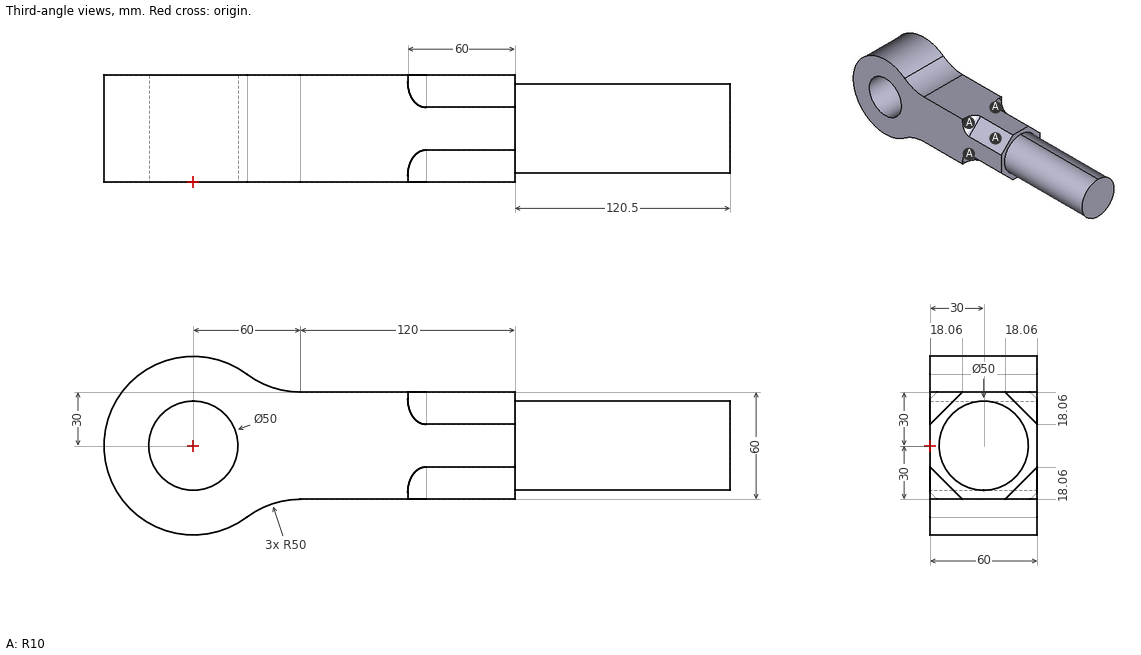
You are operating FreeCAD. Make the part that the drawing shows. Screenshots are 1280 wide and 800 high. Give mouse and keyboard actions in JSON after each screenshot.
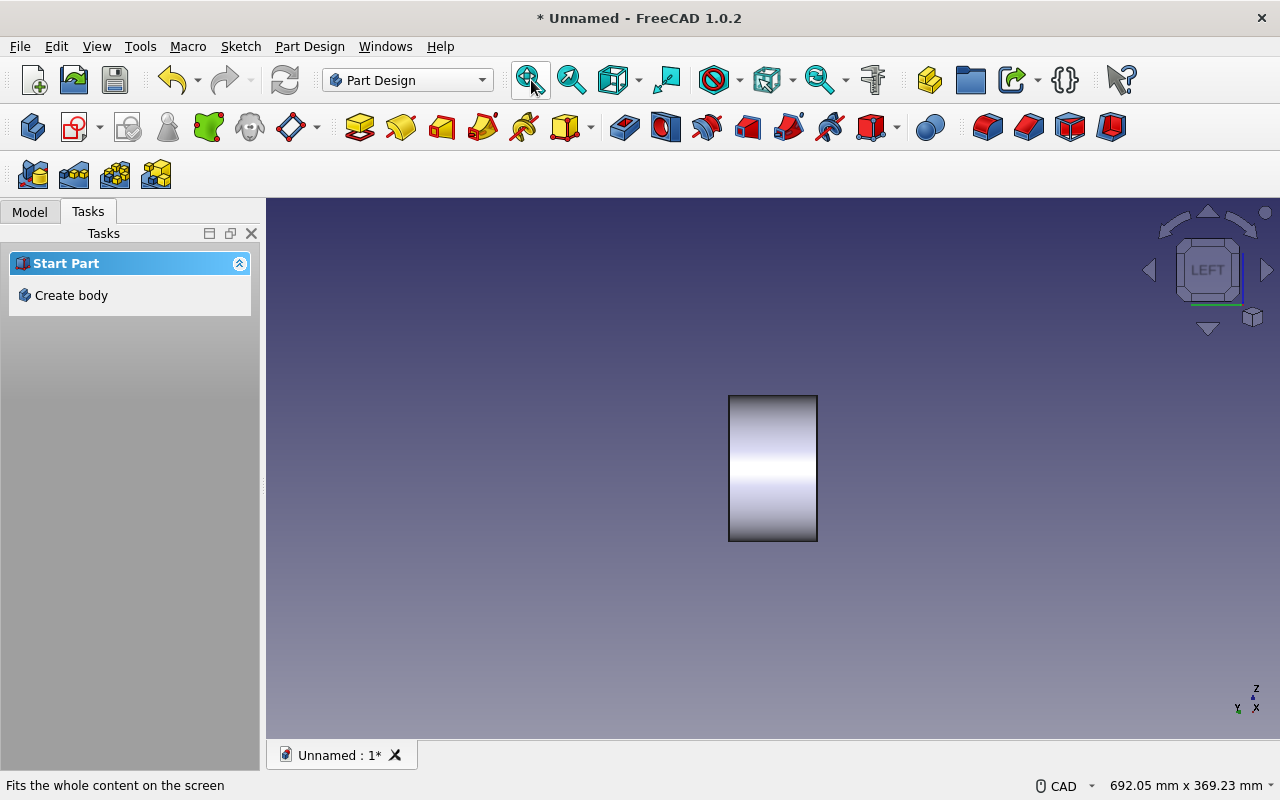
{"action": "key", "text": "v 3"}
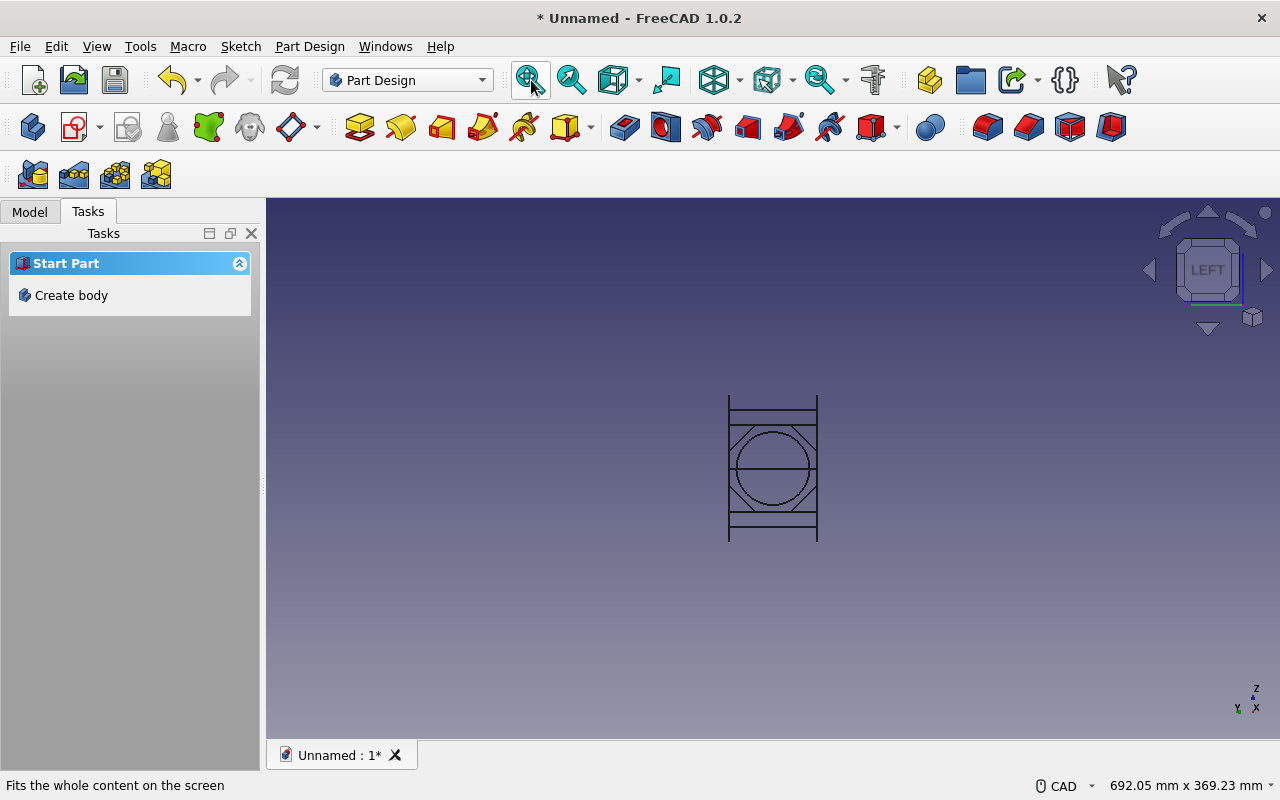
{"action": "key", "text": "0"}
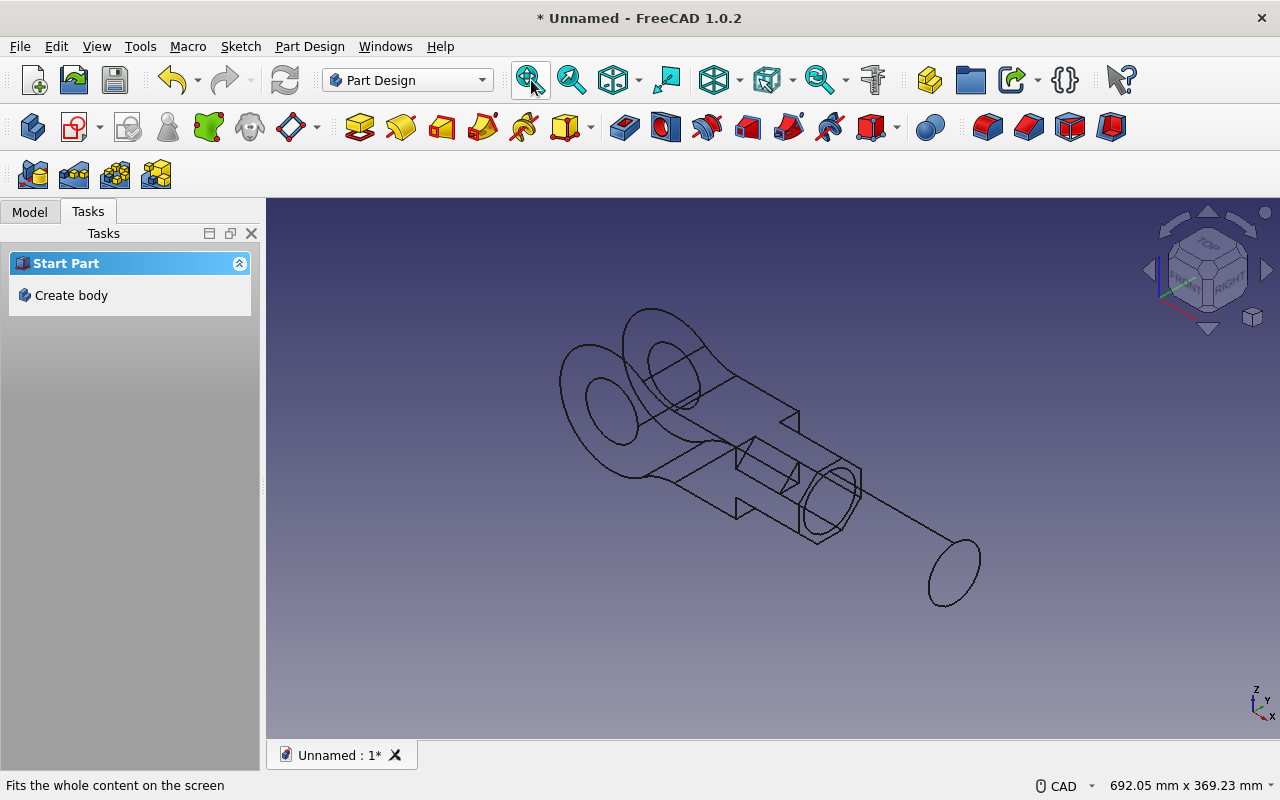
{"action": "left_click", "coordinate": [789, 477]}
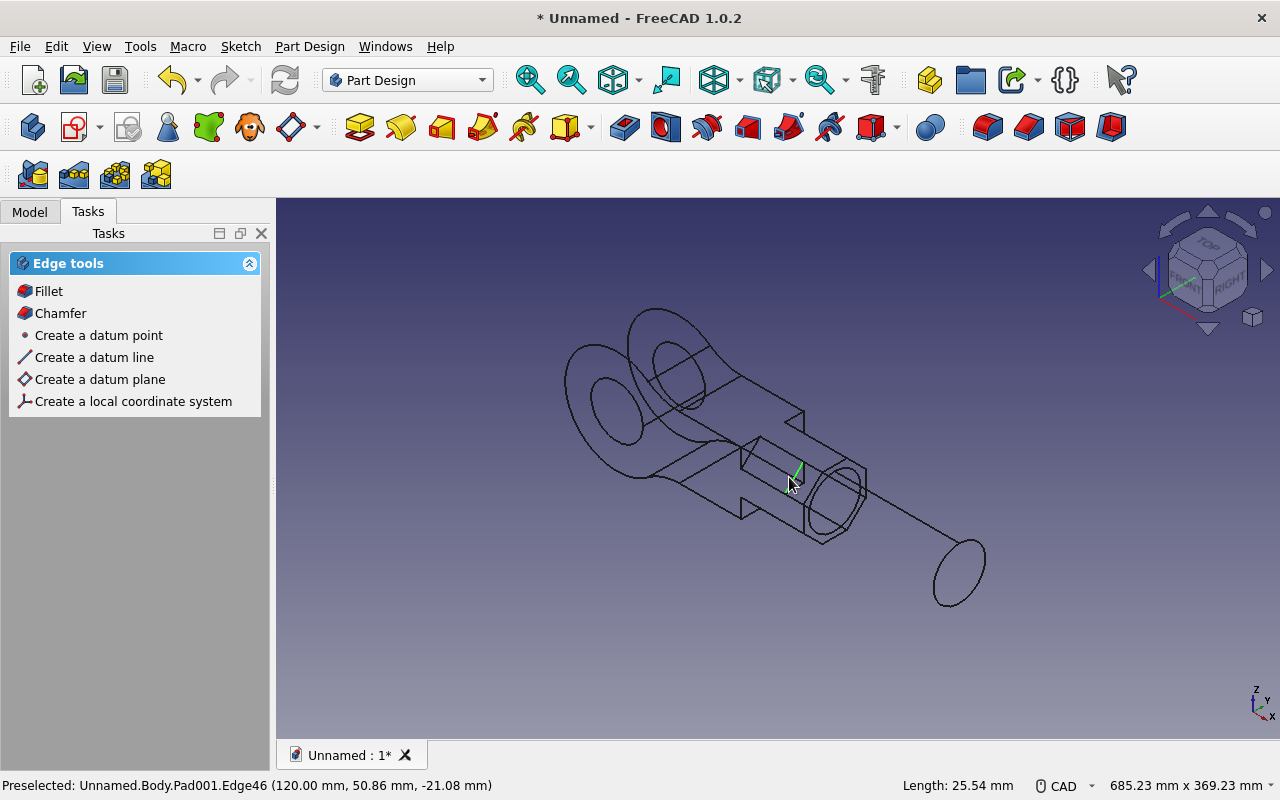
{"action": "left_click", "coordinate": [751, 452], "text": "ctrl"}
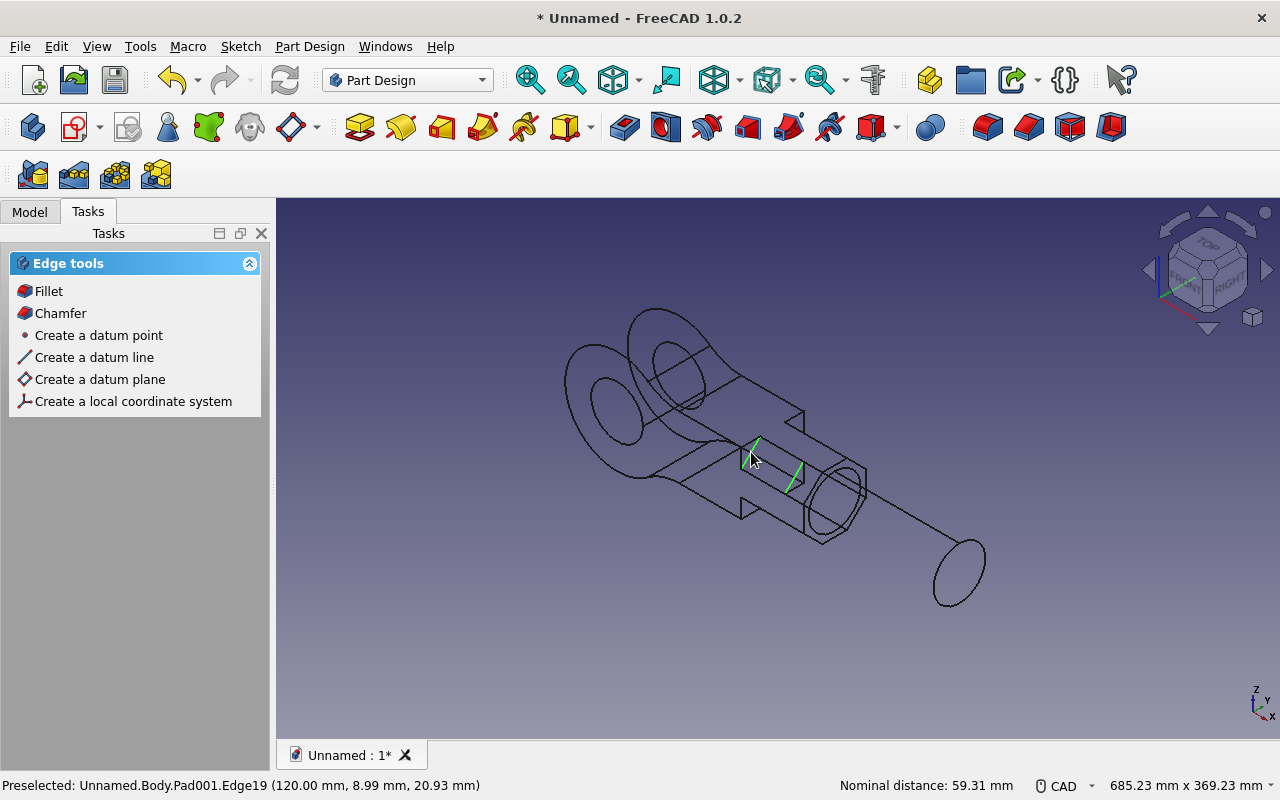
{"action": "key", "text": "2"}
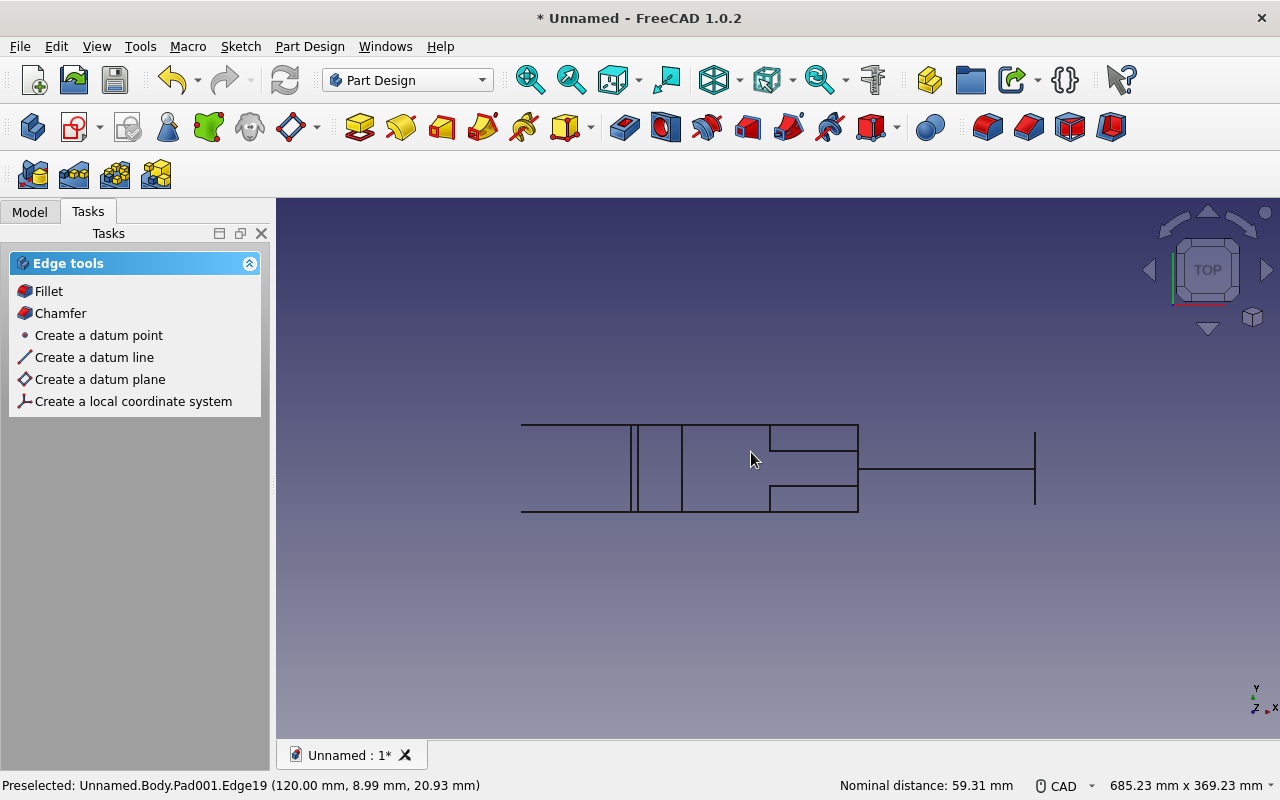
{"action": "key", "text": "1"}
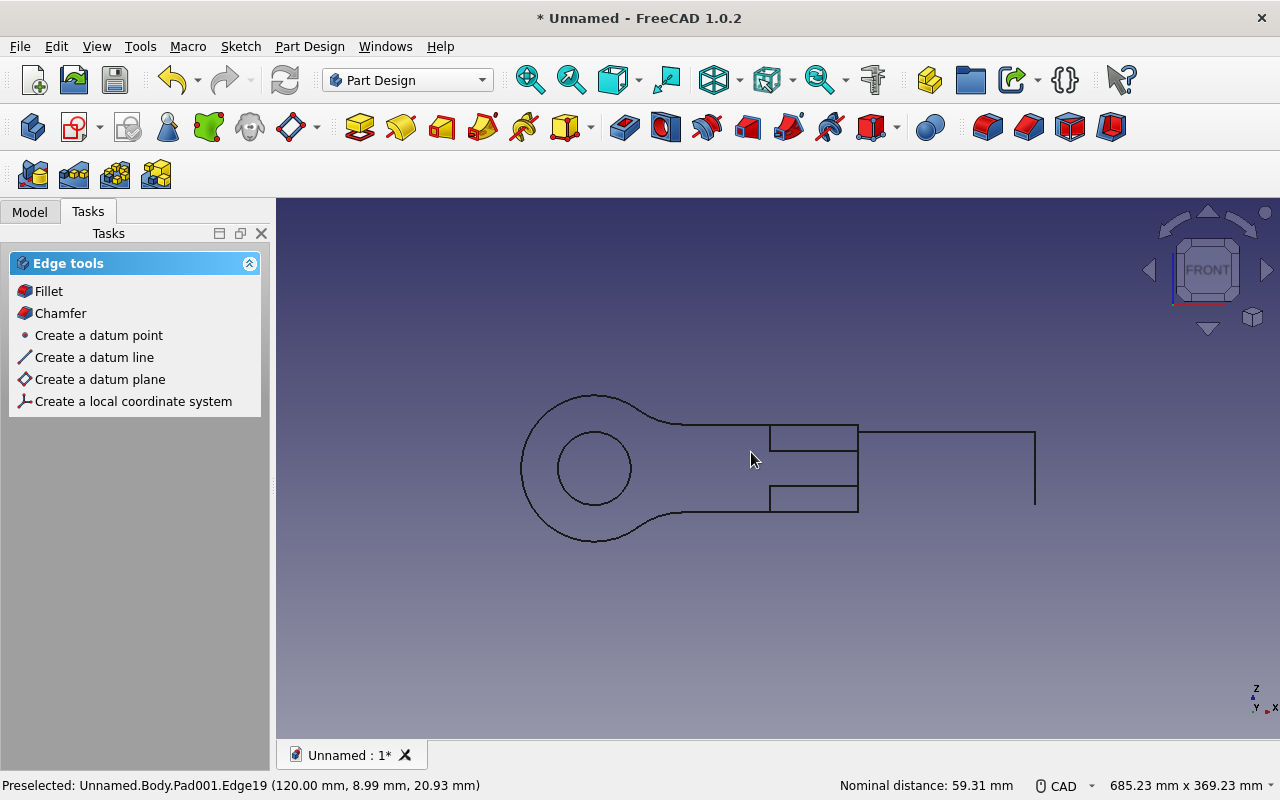
{"action": "key", "text": "3"}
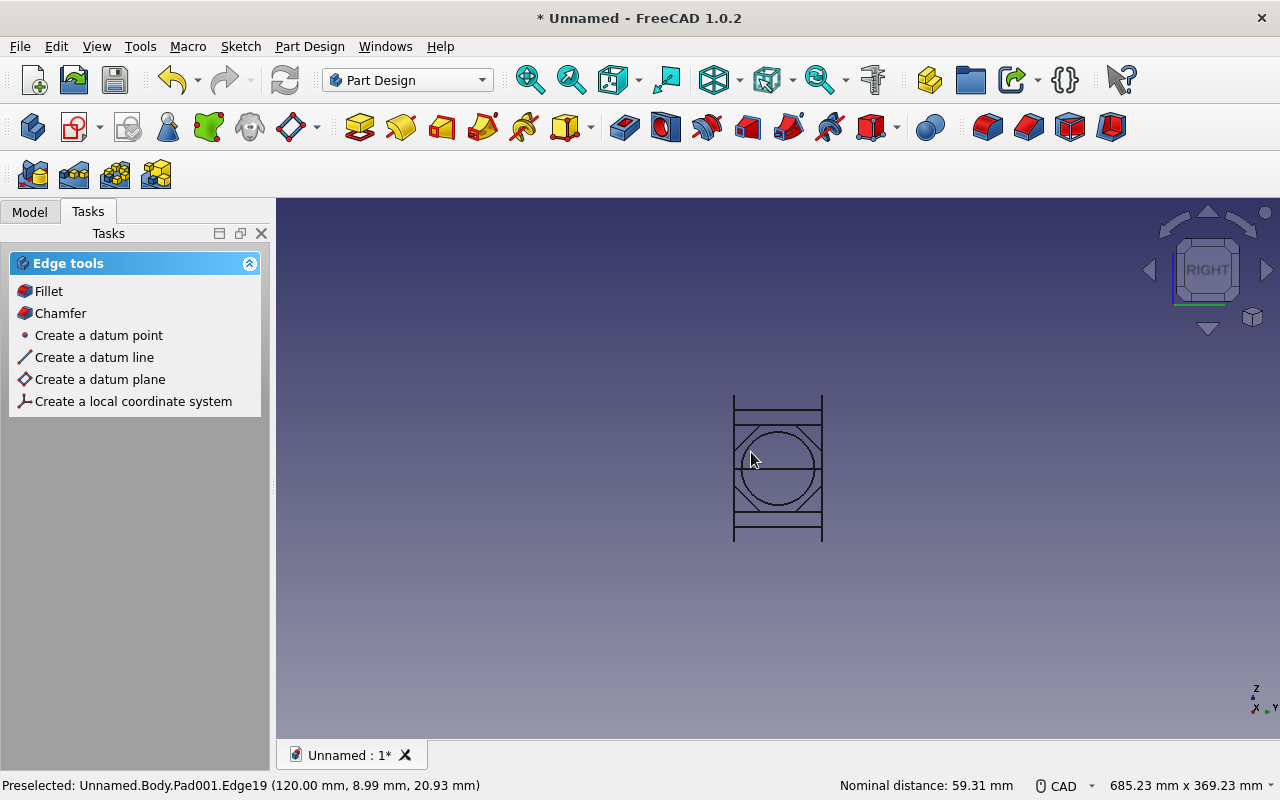
{"action": "key", "text": "v f"}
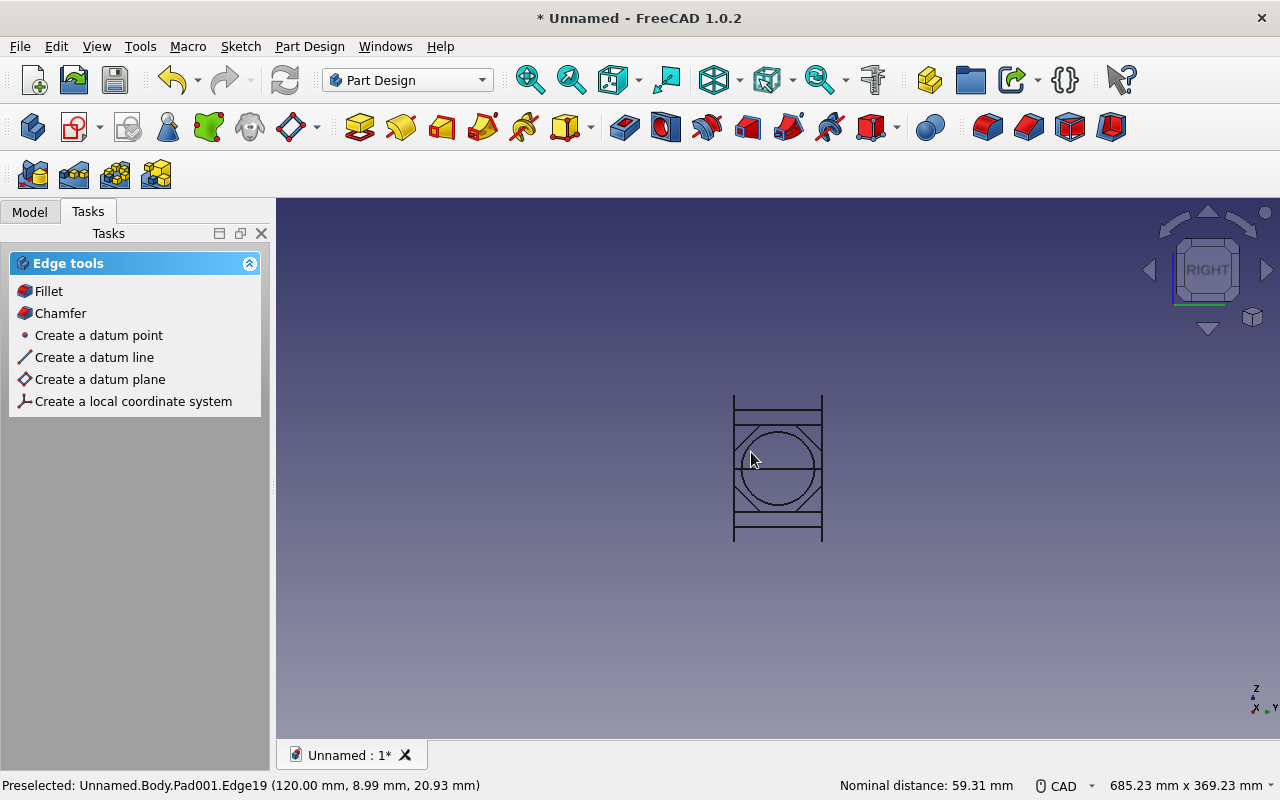
{"action": "key", "text": "5"}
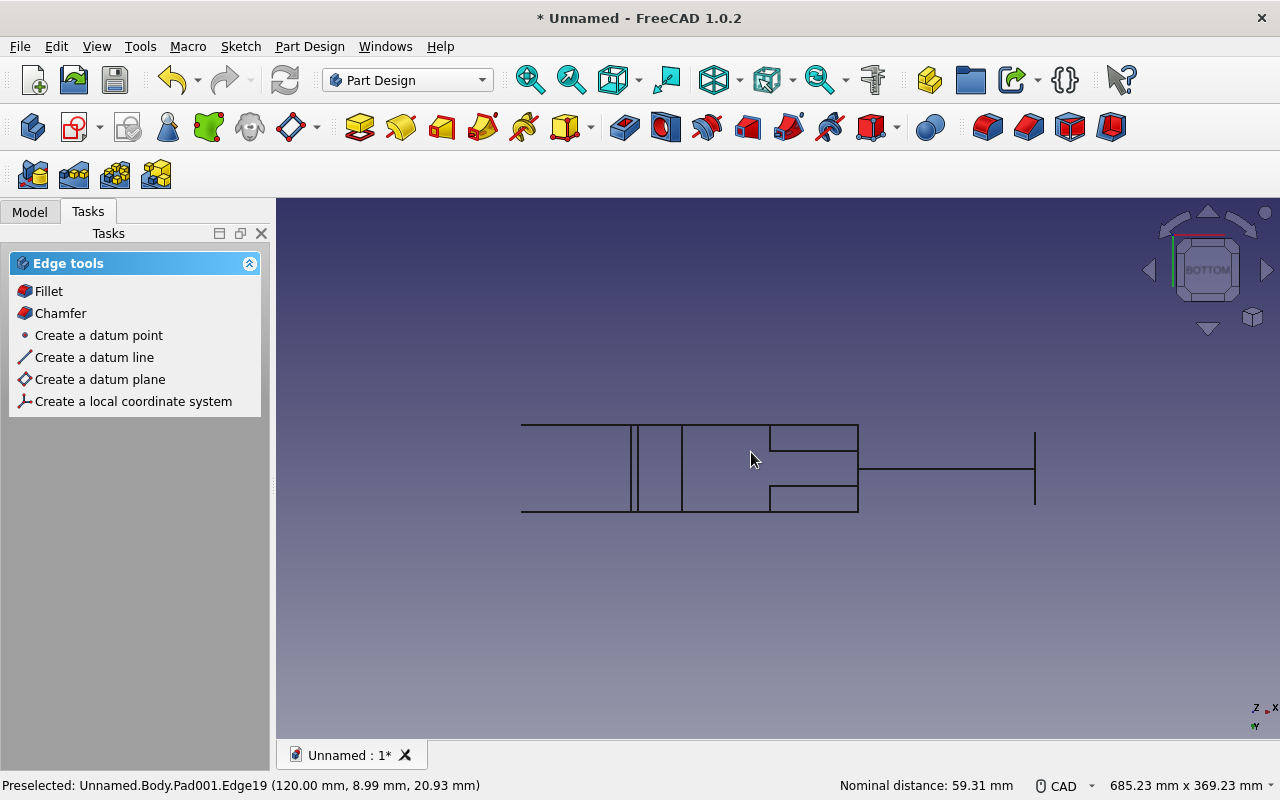
{"action": "key", "text": "4"}